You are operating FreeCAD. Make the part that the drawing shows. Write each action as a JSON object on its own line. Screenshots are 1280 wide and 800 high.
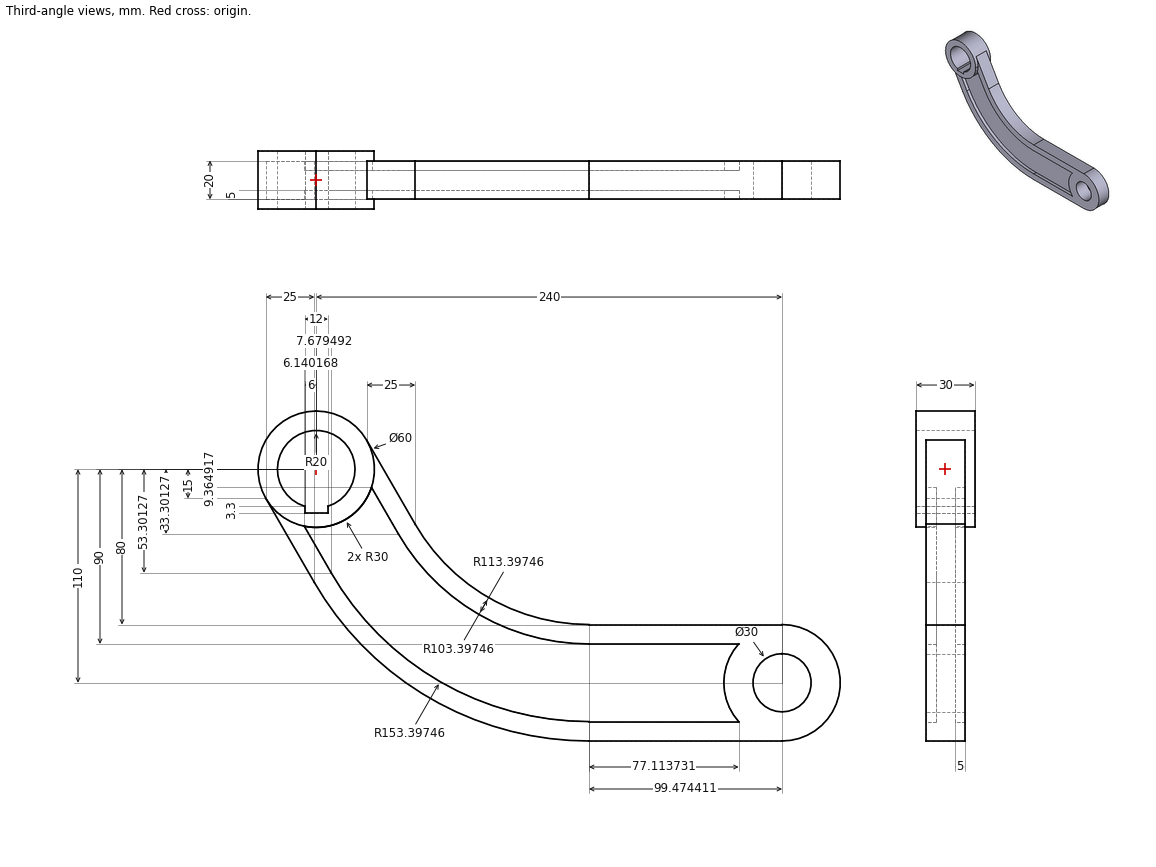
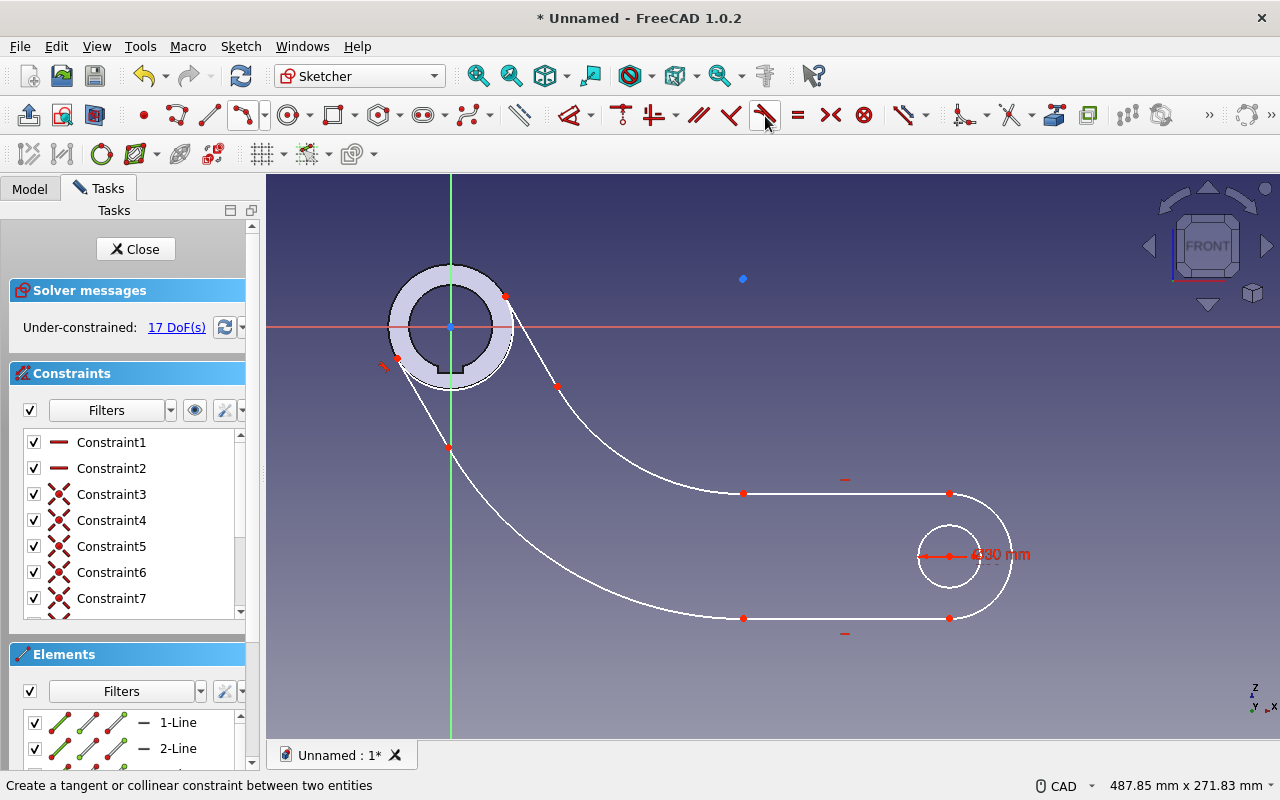
{"action": "left_click", "coordinate": [541, 360]}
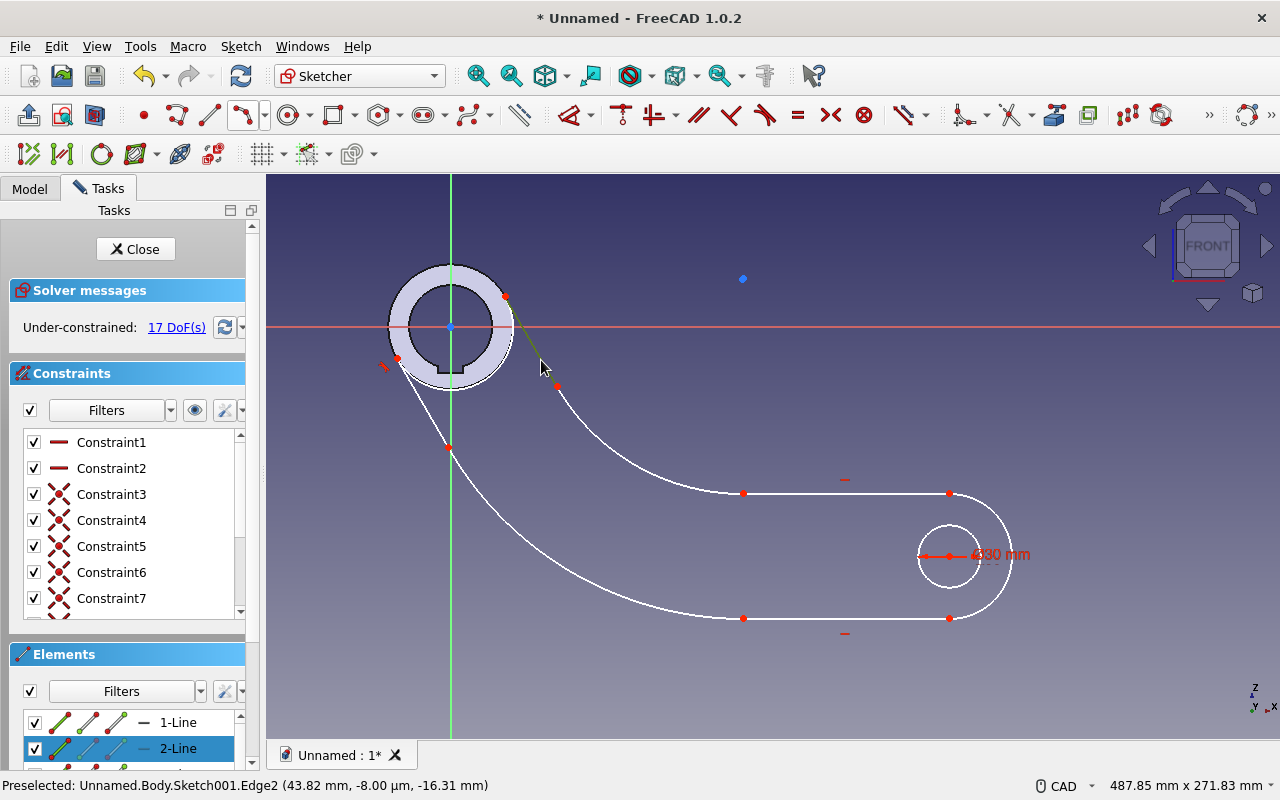
{"action": "left_click", "coordinate": [508, 353]}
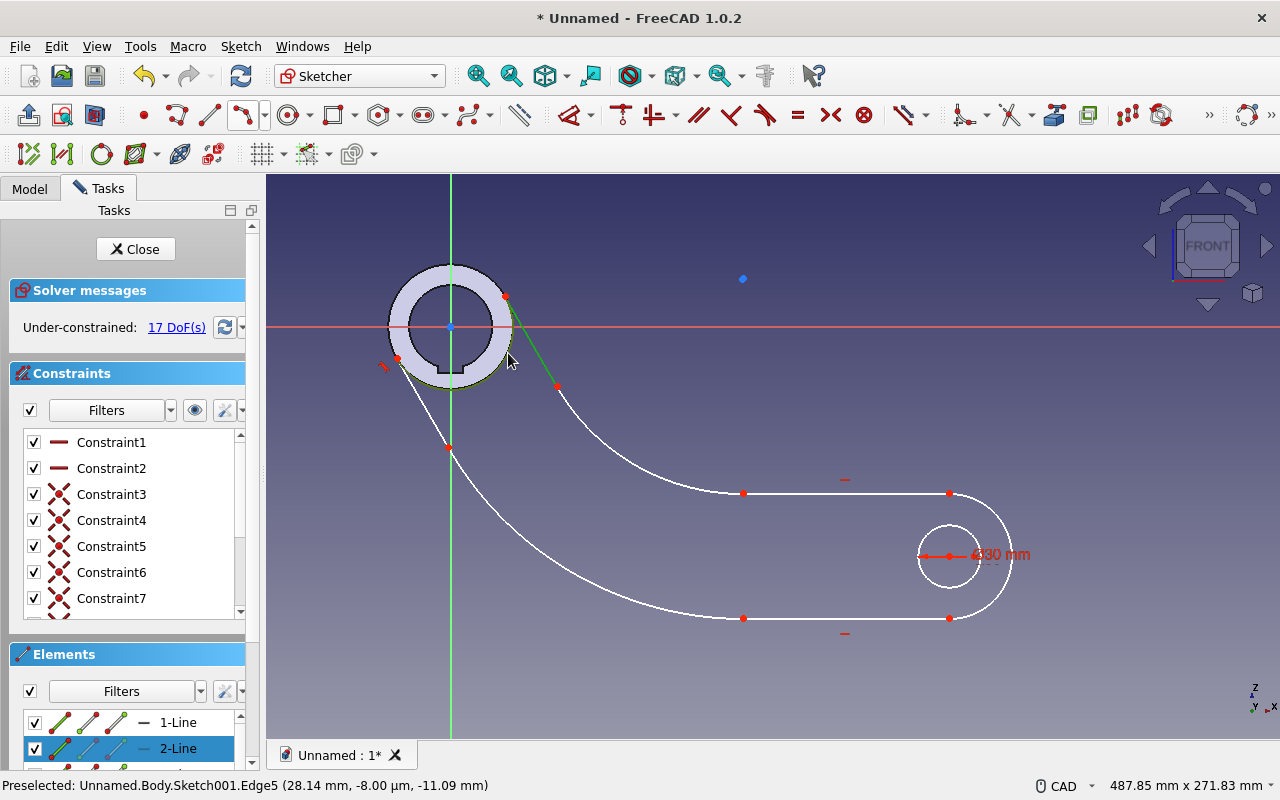
{"action": "key", "text": "t"}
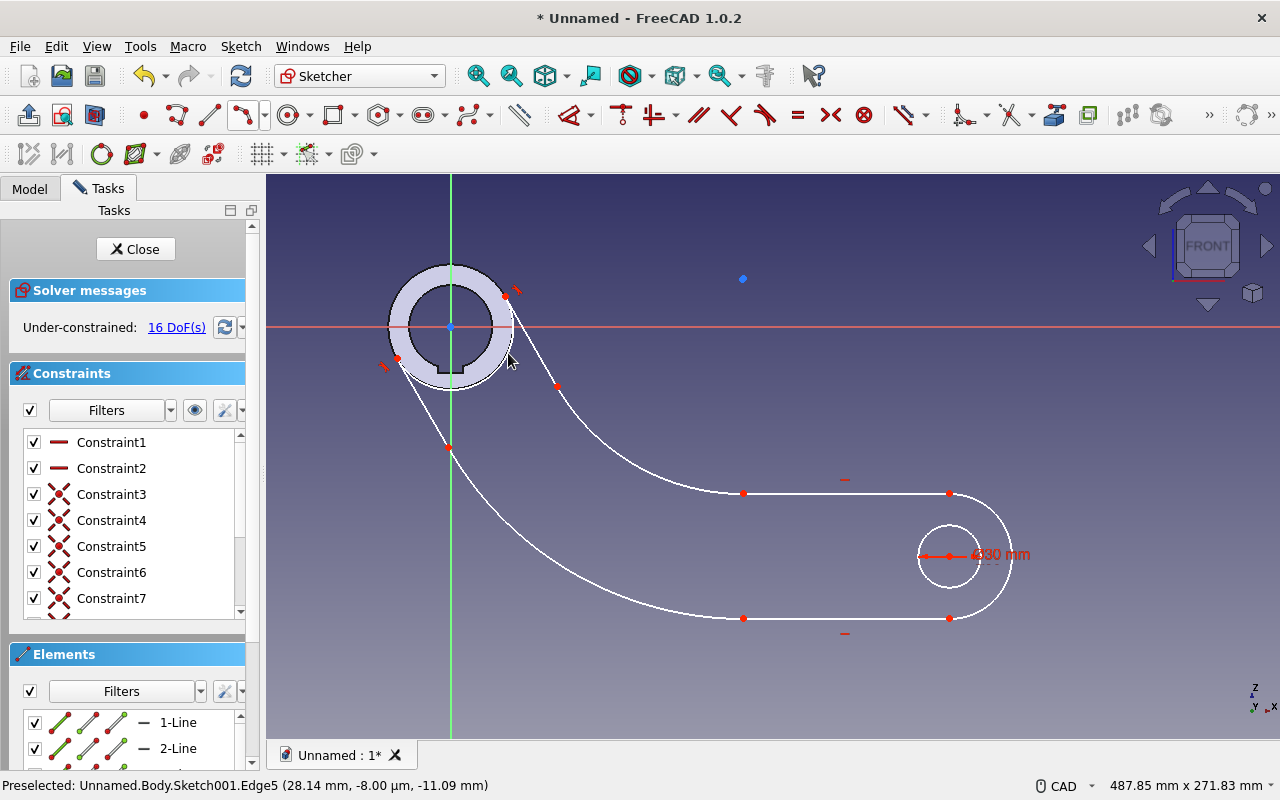
{"action": "left_click", "coordinate": [805, 494]}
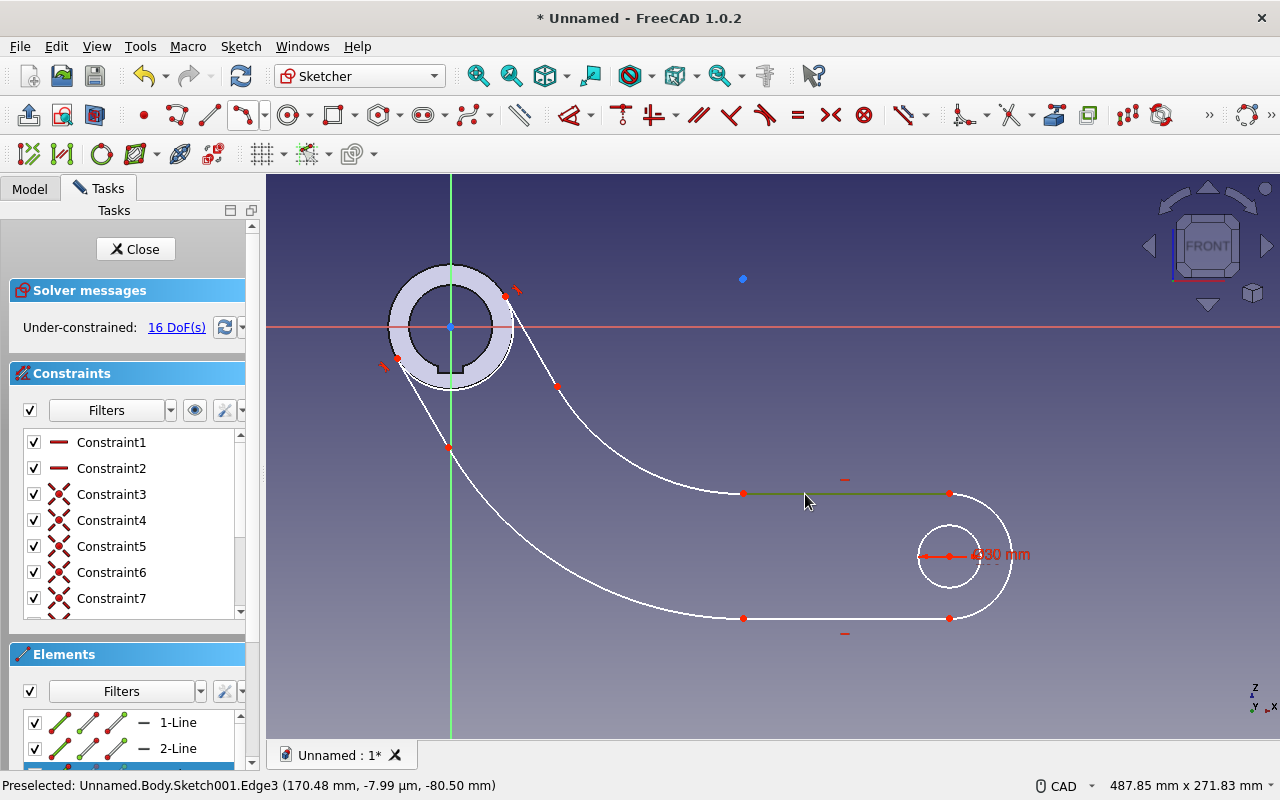
{"action": "left_click", "coordinate": [1000, 593]}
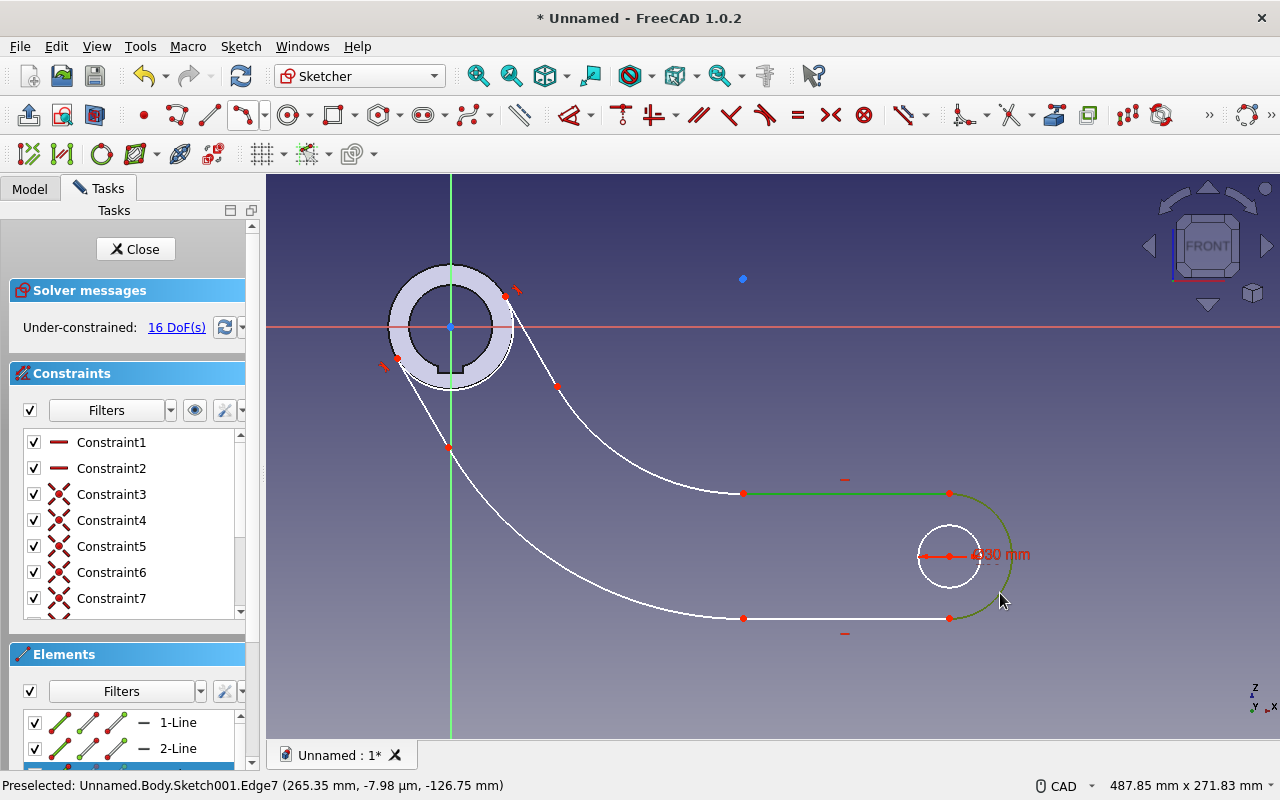
{"action": "left_click", "coordinate": [765, 116]}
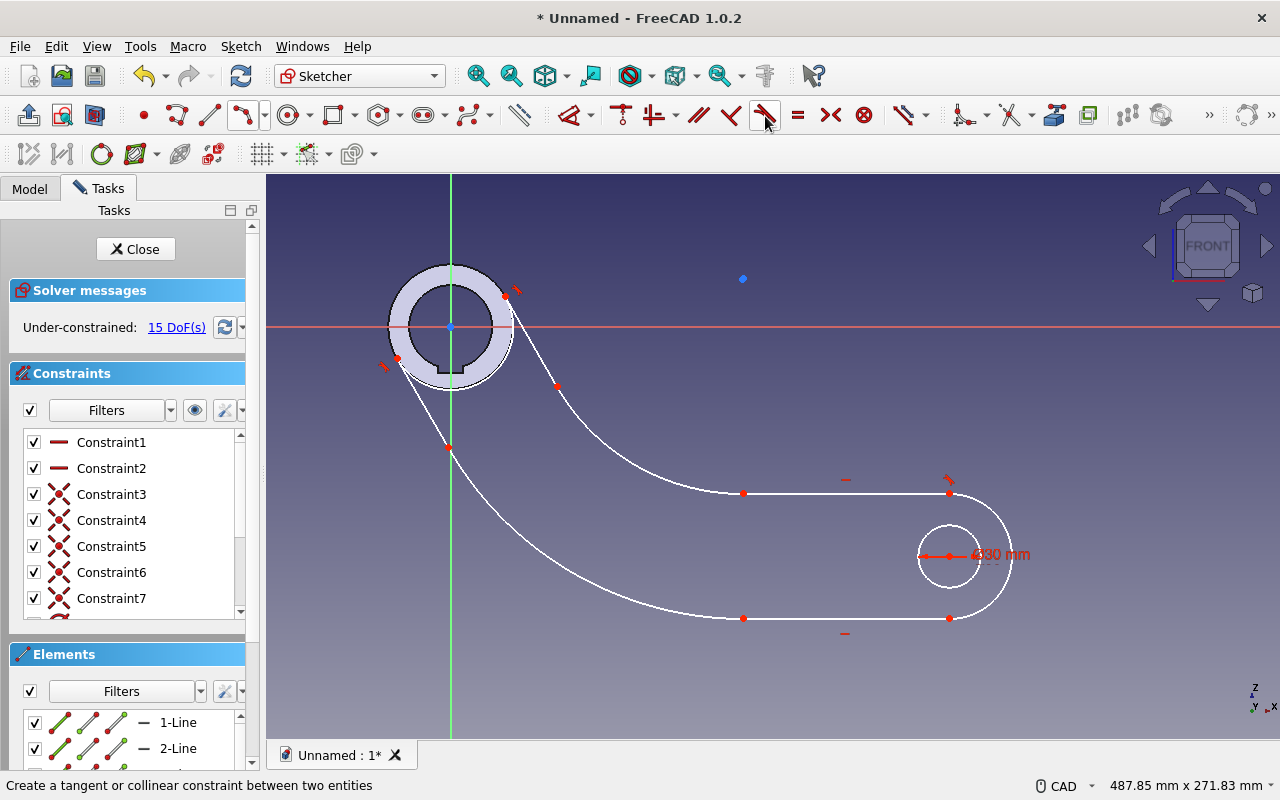
{"action": "left_click", "coordinate": [887, 619]}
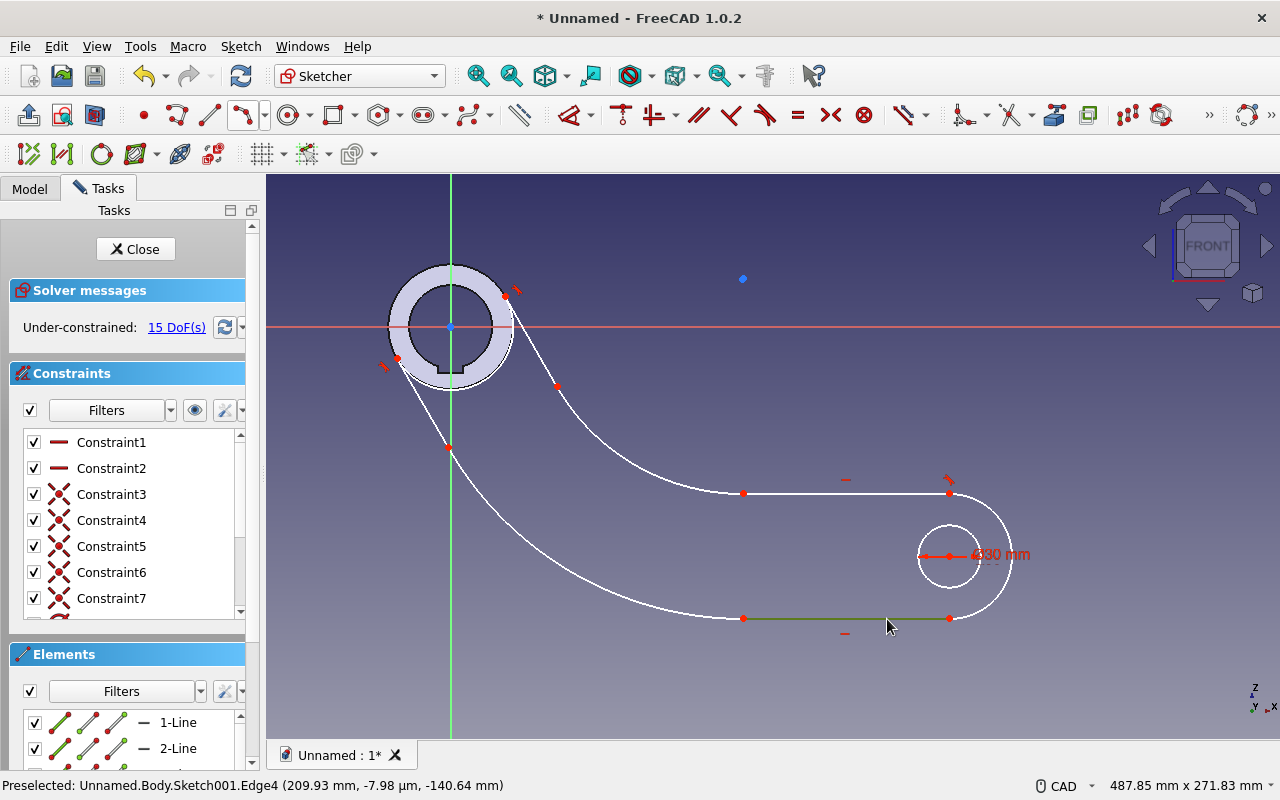
{"action": "left_click", "coordinate": [1000, 594]}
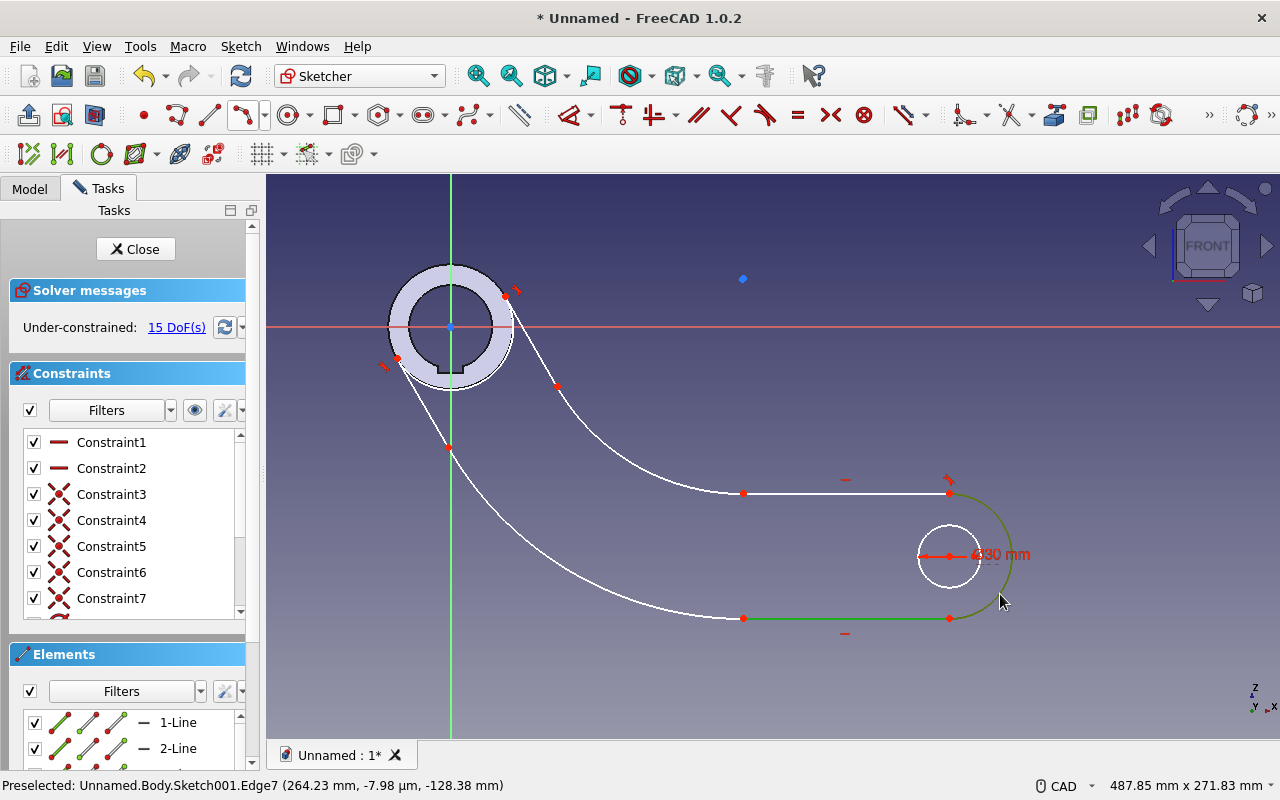
{"action": "left_click", "coordinate": [765, 116]}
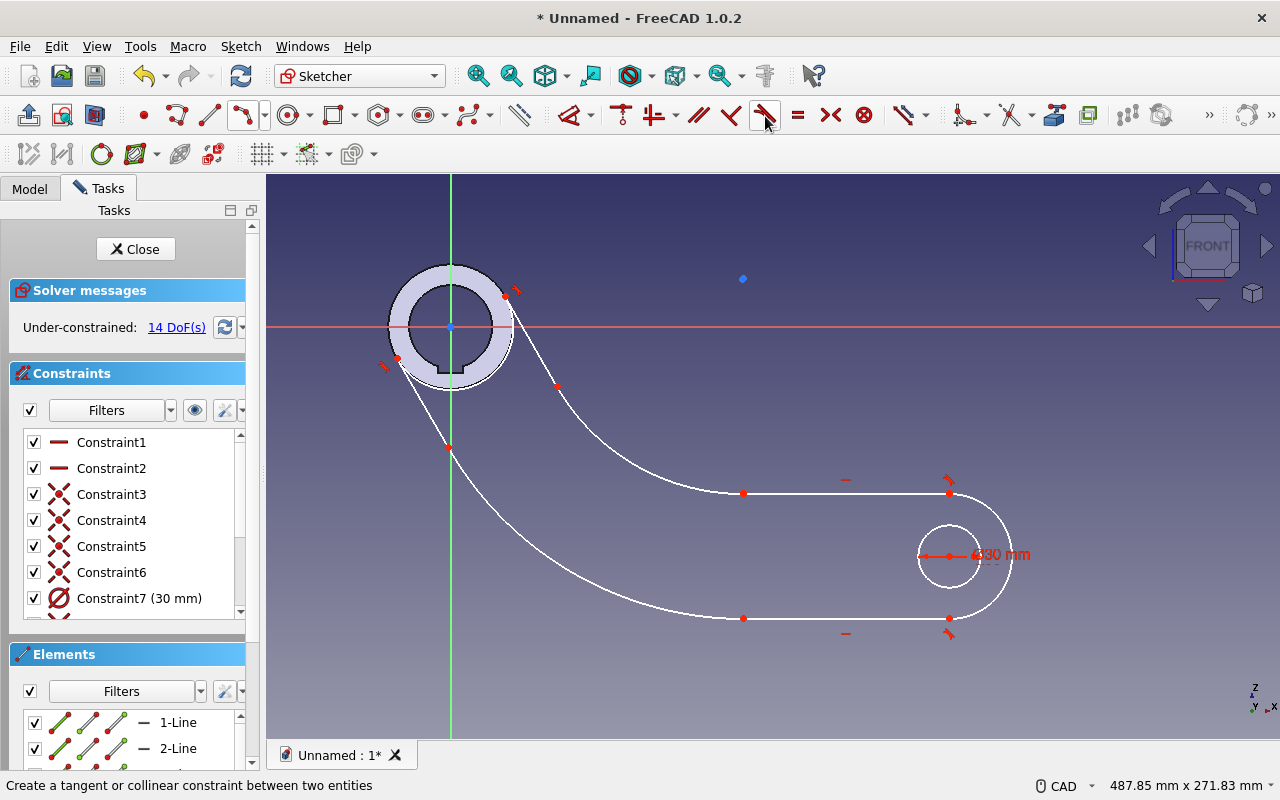
{"action": "left_click", "coordinate": [599, 439]}